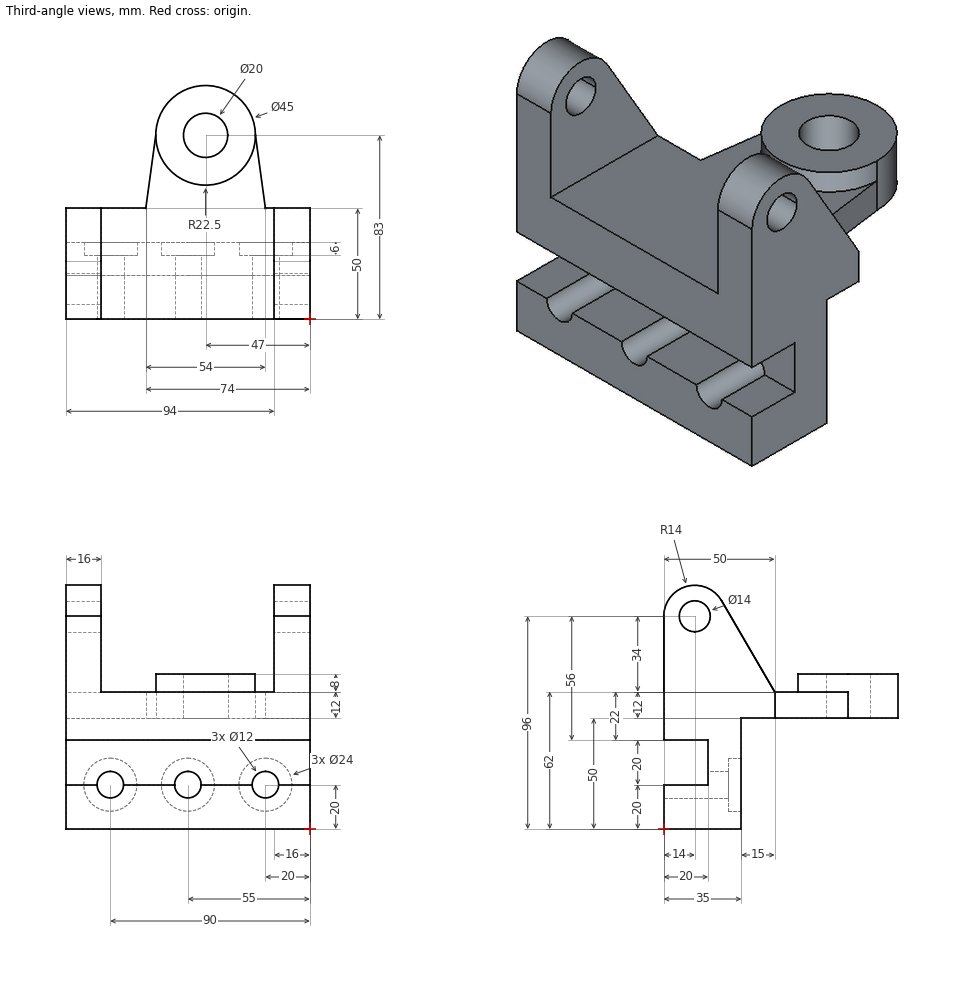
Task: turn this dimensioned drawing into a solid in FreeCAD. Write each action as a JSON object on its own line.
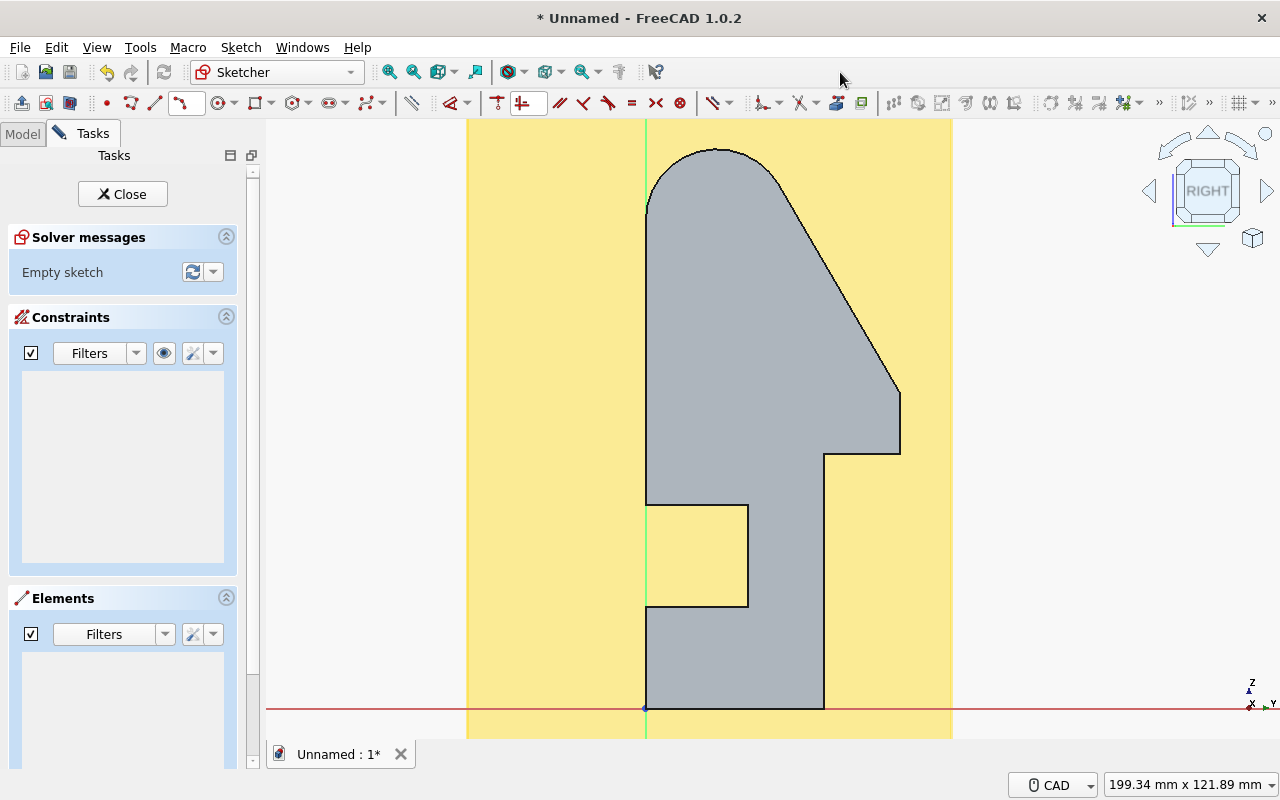
{"action": "left_click", "coordinate": [70, 104]}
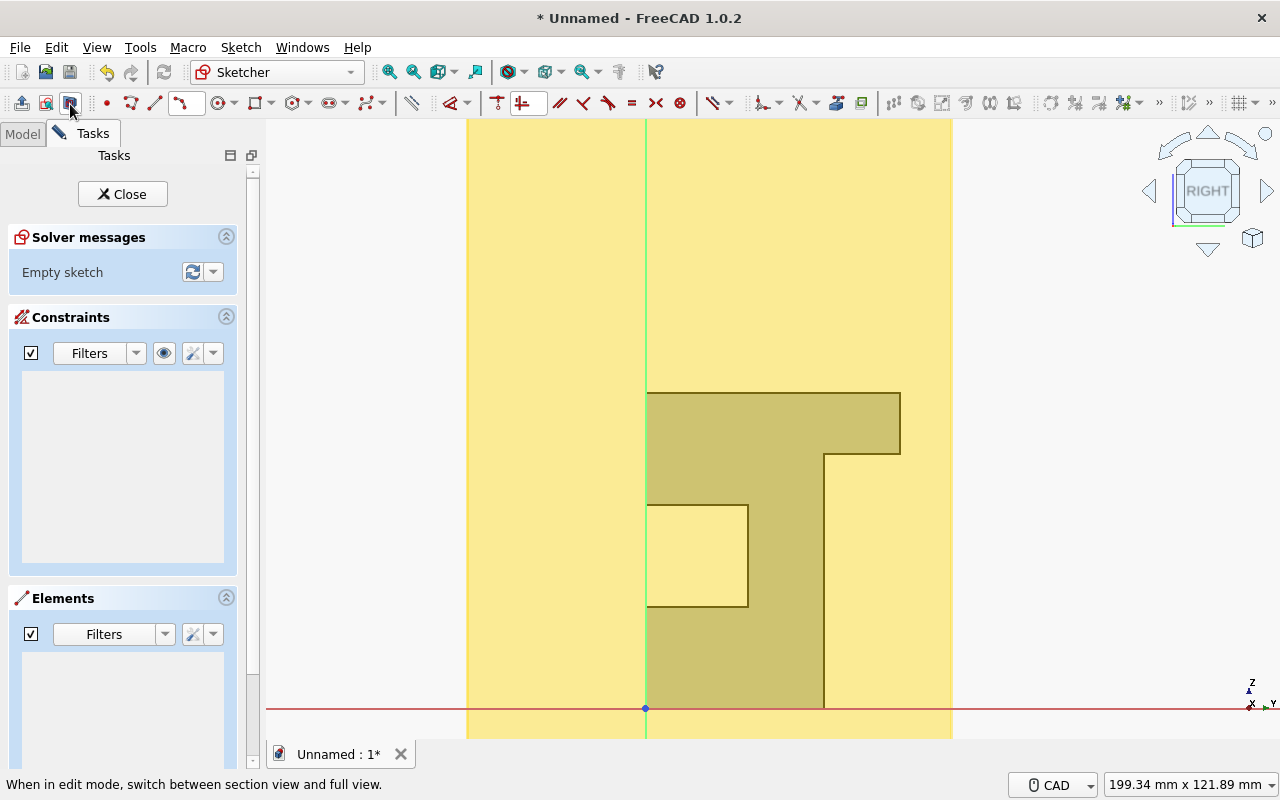
{"action": "scroll", "coordinate": [565, 426], "scroll_direction": "down", "scroll_amount": 2}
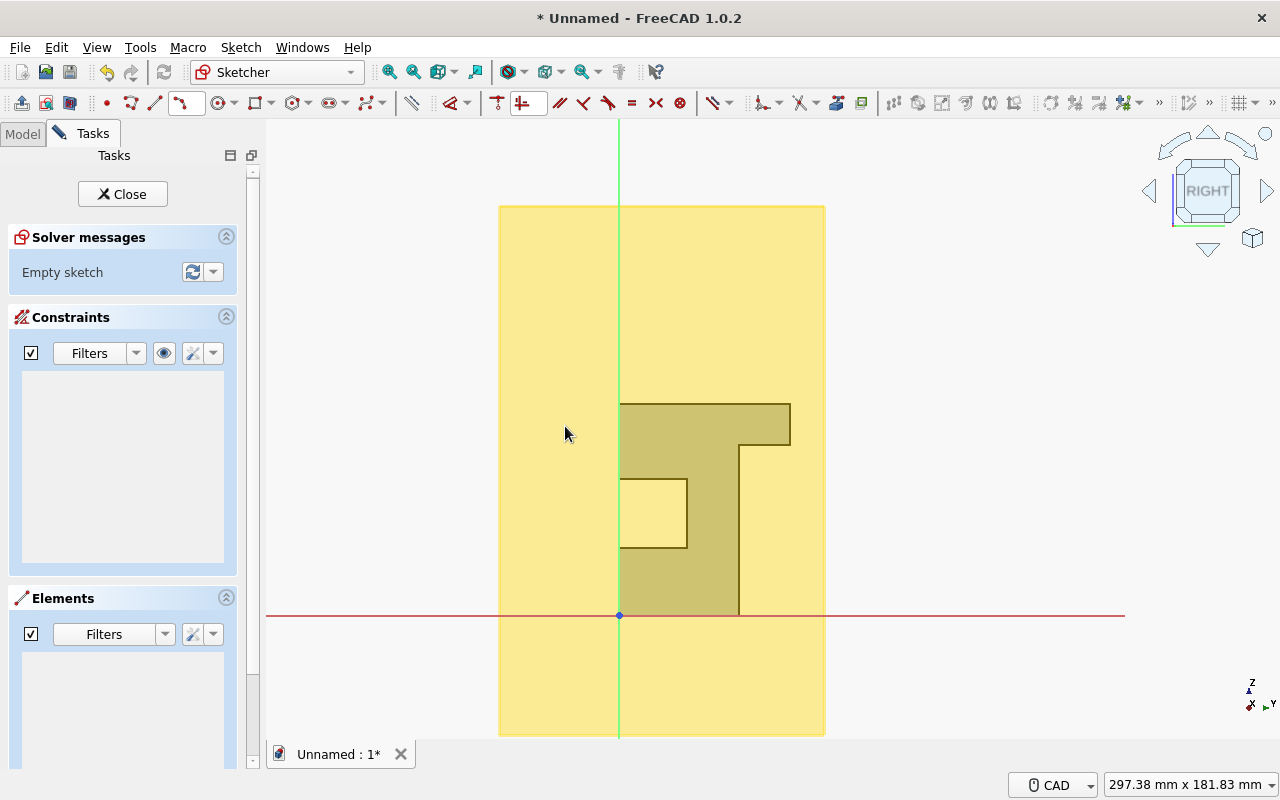
{"action": "left_click", "coordinate": [132, 104]}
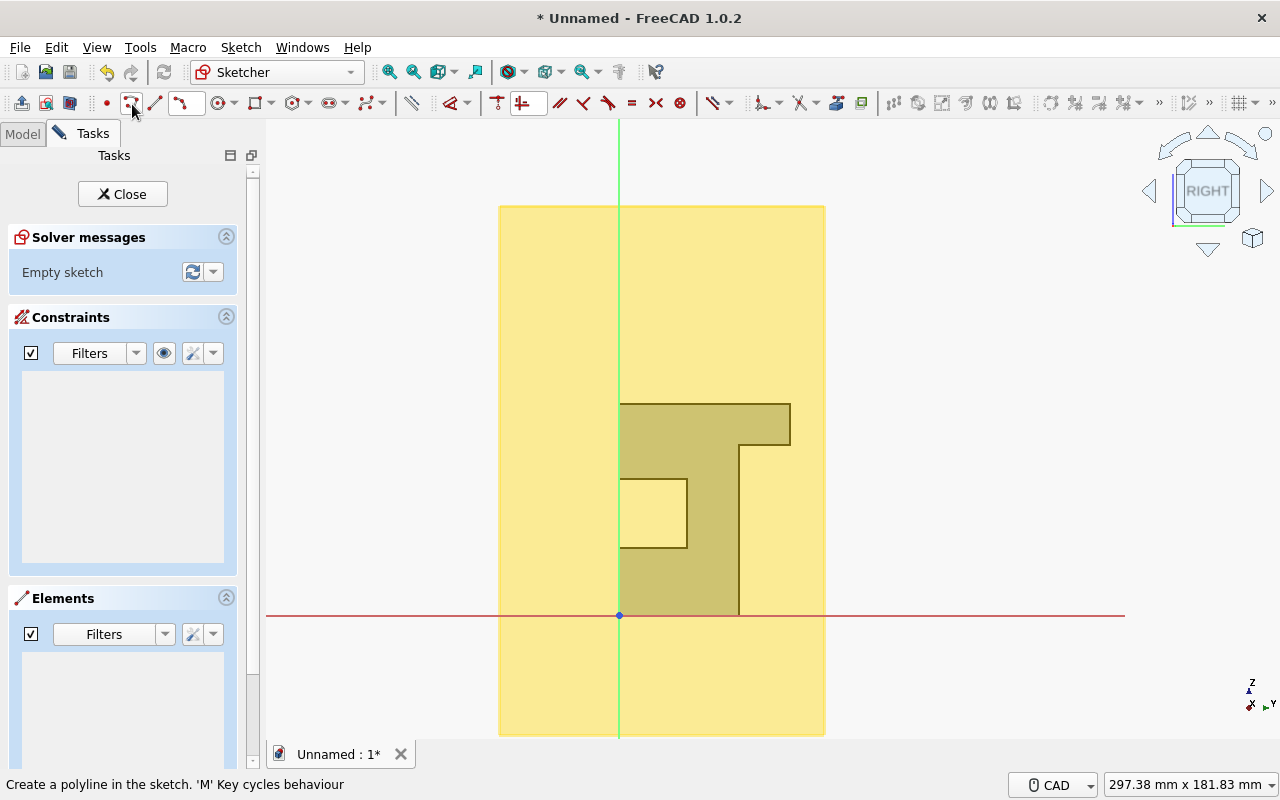
{"action": "left_click", "coordinate": [708, 264]}
{"action": "left_click", "coordinate": [790, 404]}
{"action": "left_click", "coordinate": [619, 404]}
{"action": "left_click", "coordinate": [628, 288]}
{"action": "right_click", "coordinate": [628, 288]}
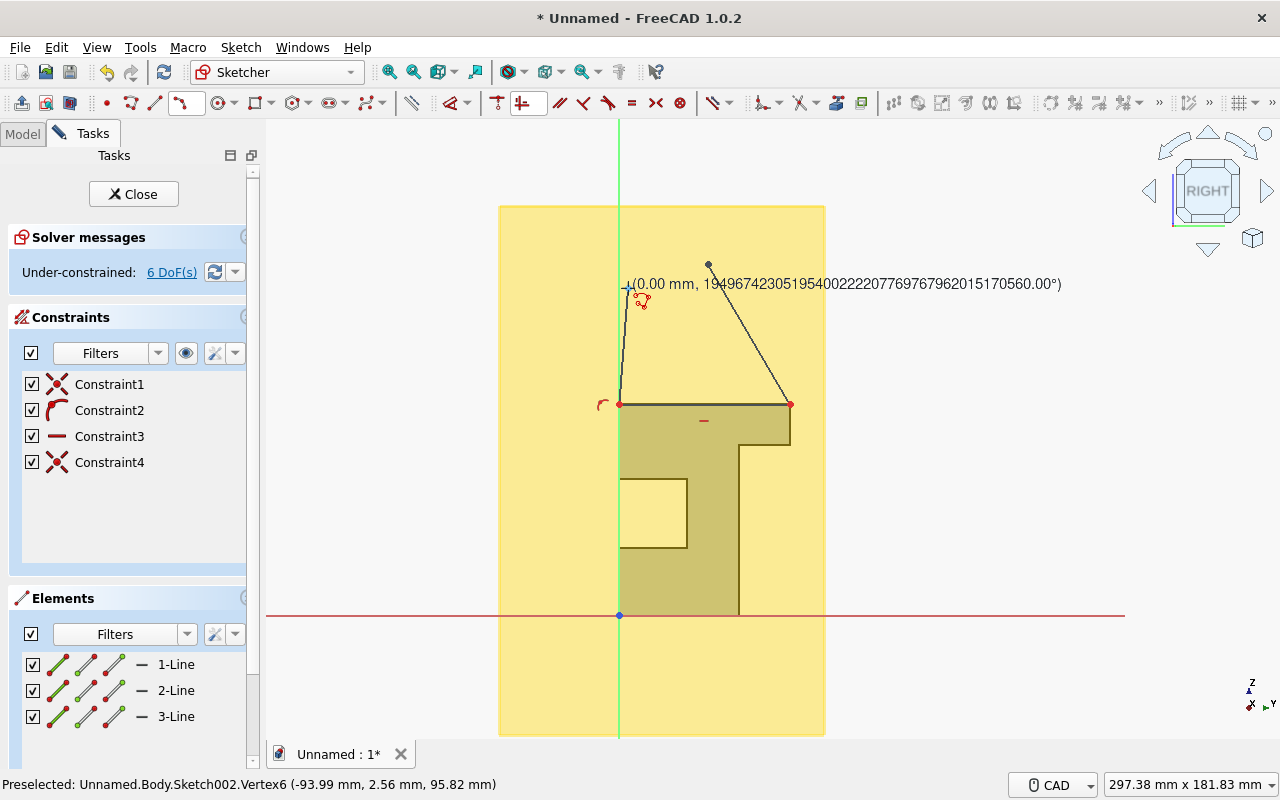
{"action": "left_click", "coordinate": [180, 104]}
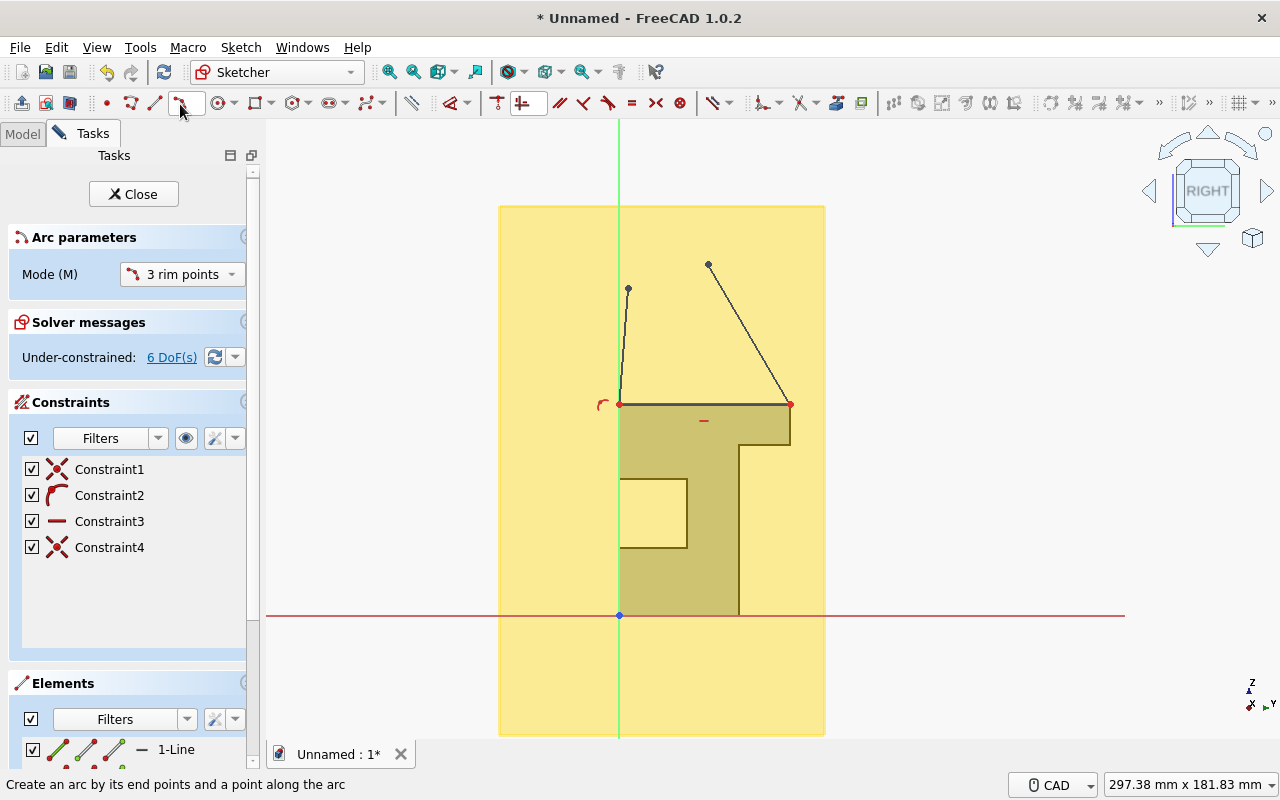
{"action": "left_click", "coordinate": [628, 289]}
{"action": "left_click", "coordinate": [708, 265]}
{"action": "left_click", "coordinate": [655, 242]}
{"action": "key", "text": "Escape"}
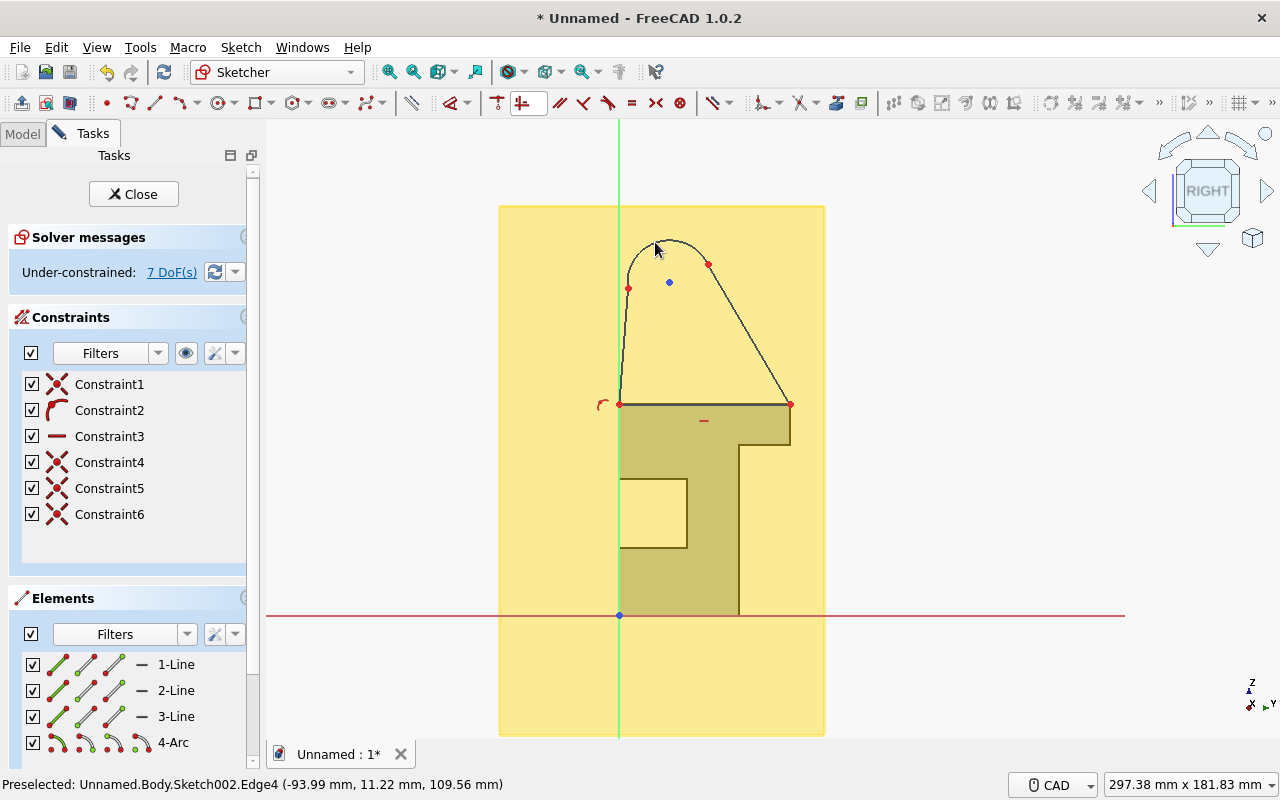
{"action": "left_click", "coordinate": [733, 307]}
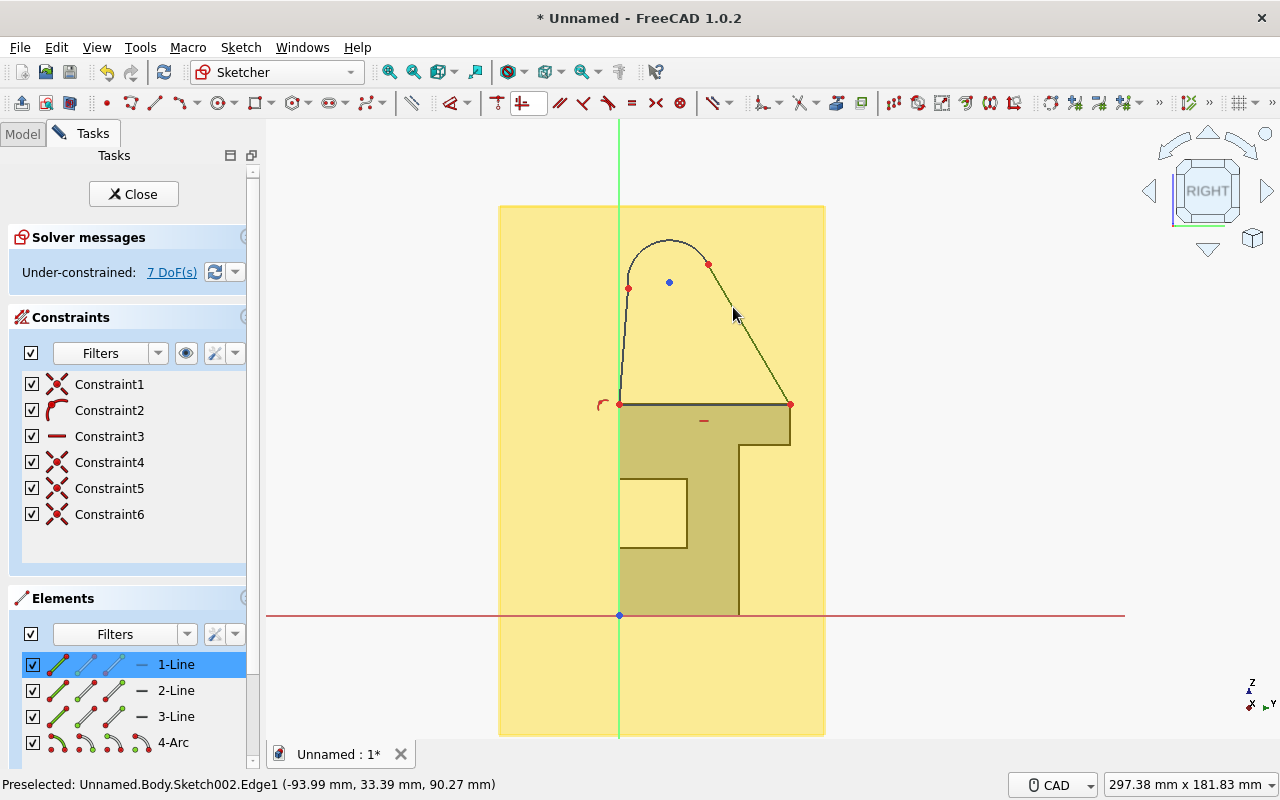
{"action": "left_click", "coordinate": [681, 242]}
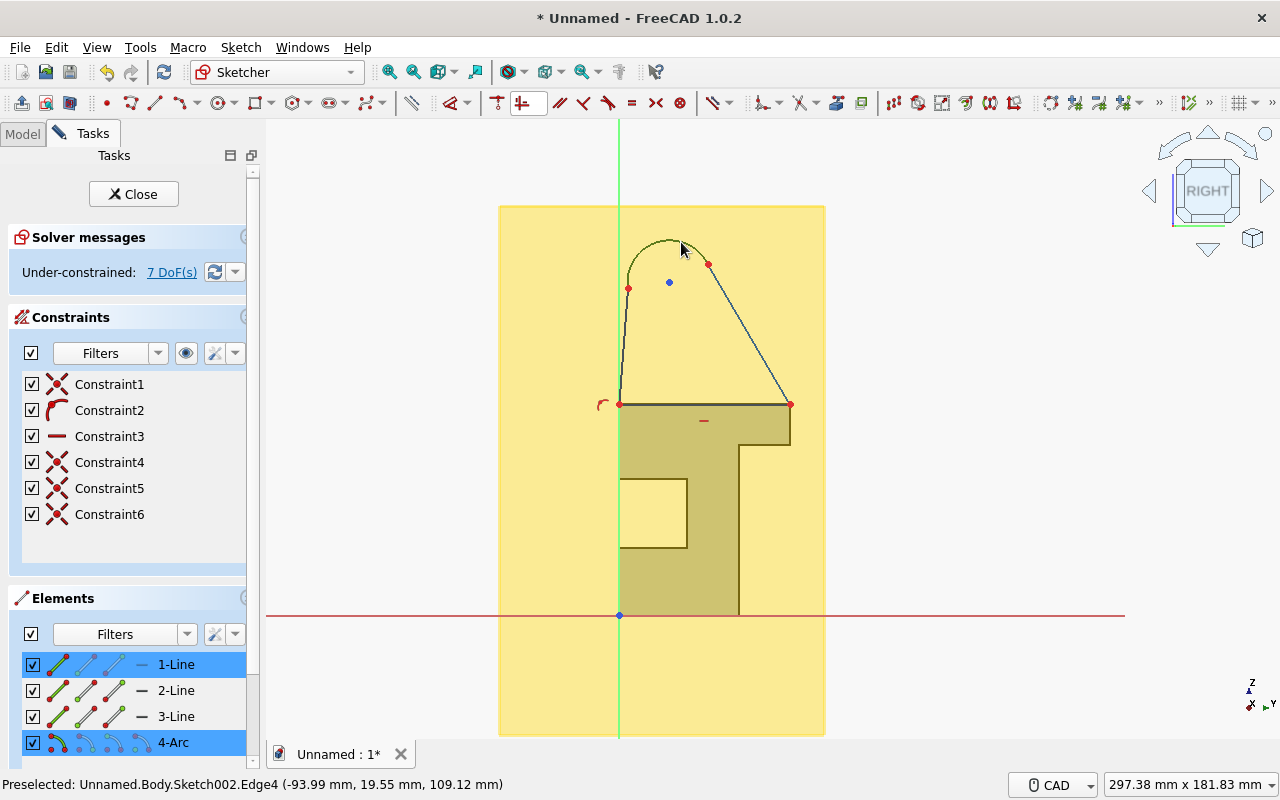
{"action": "left_click", "coordinate": [608, 104]}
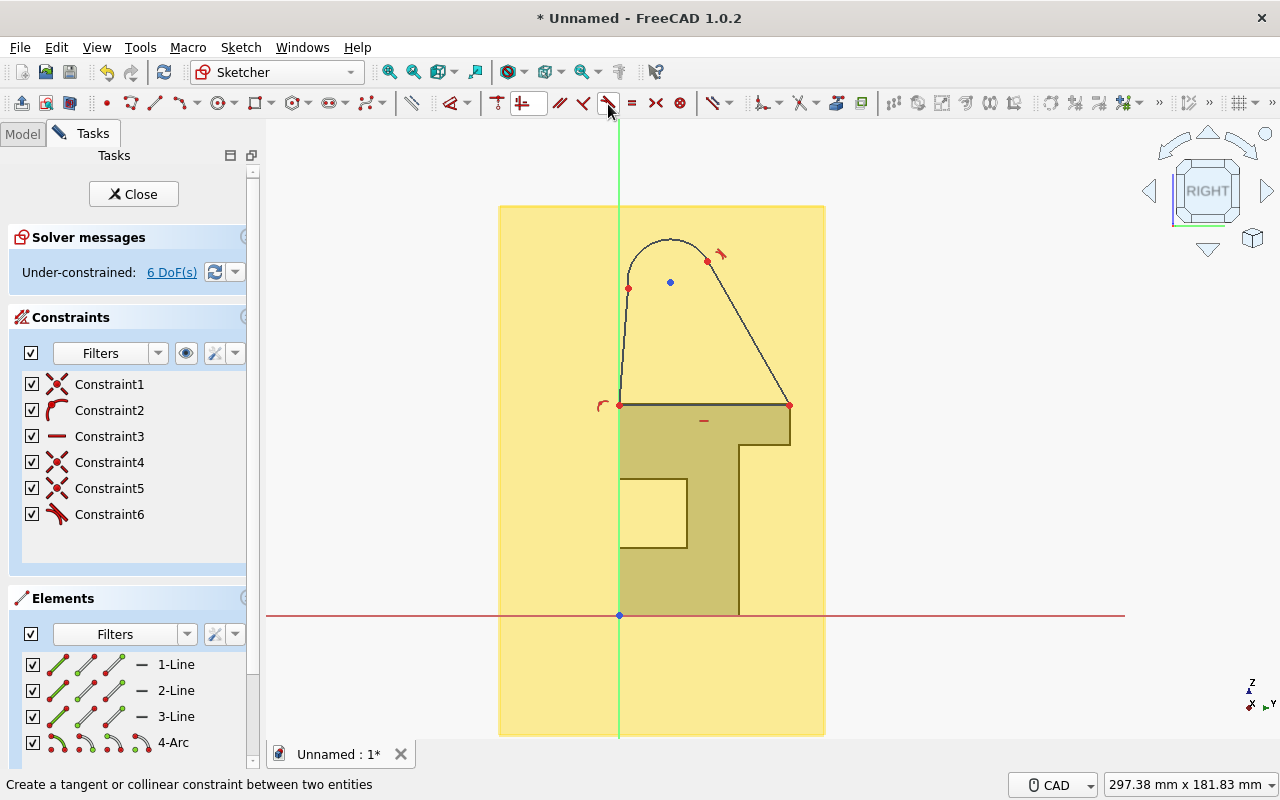
{"action": "left_click", "coordinate": [622, 370]}